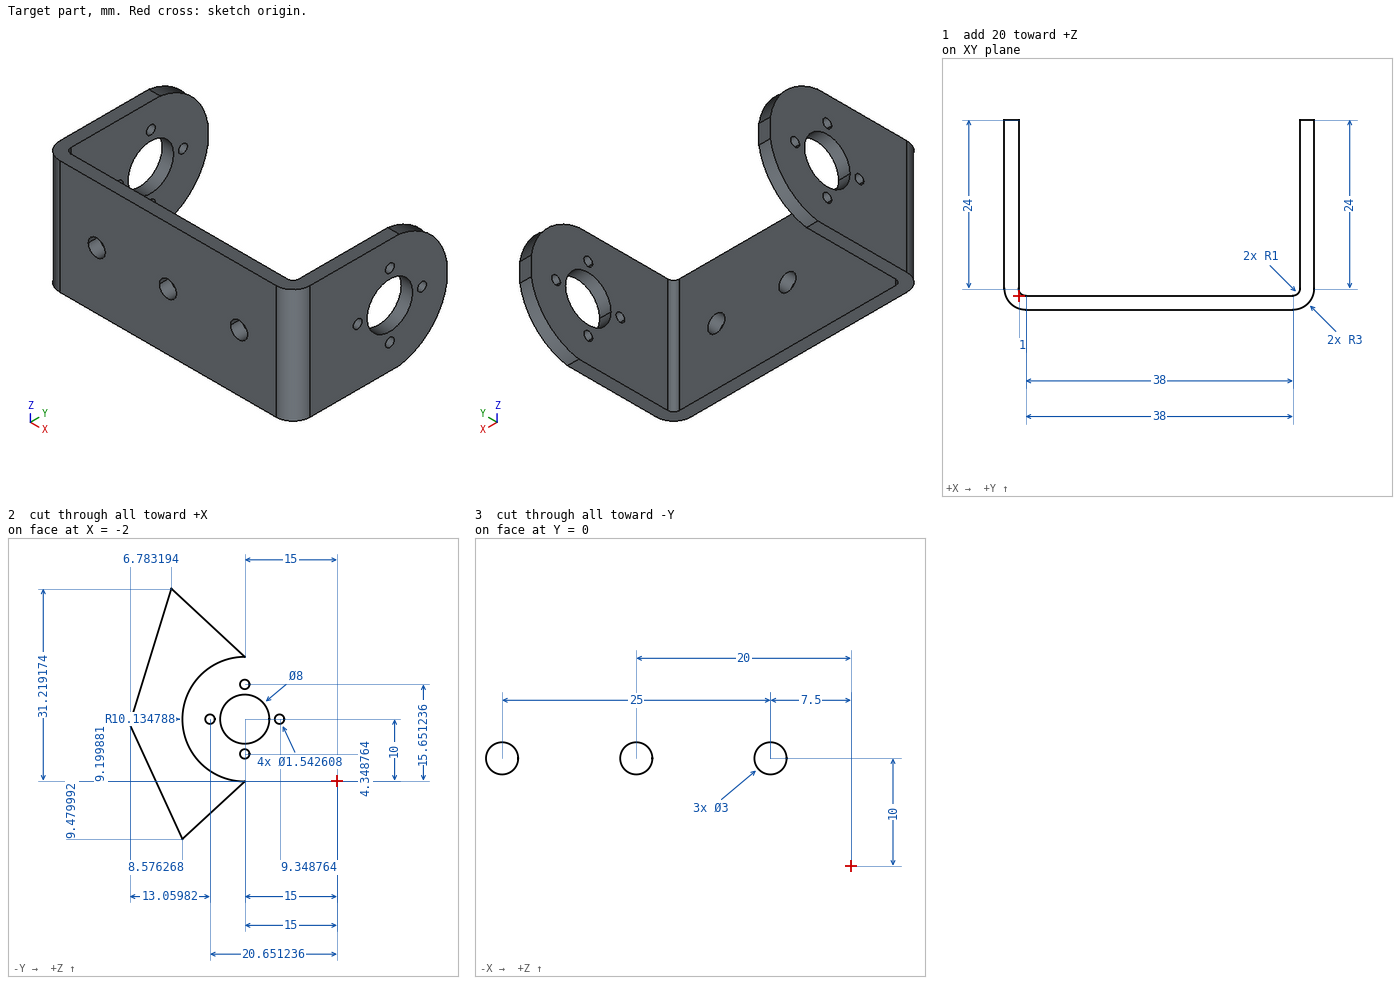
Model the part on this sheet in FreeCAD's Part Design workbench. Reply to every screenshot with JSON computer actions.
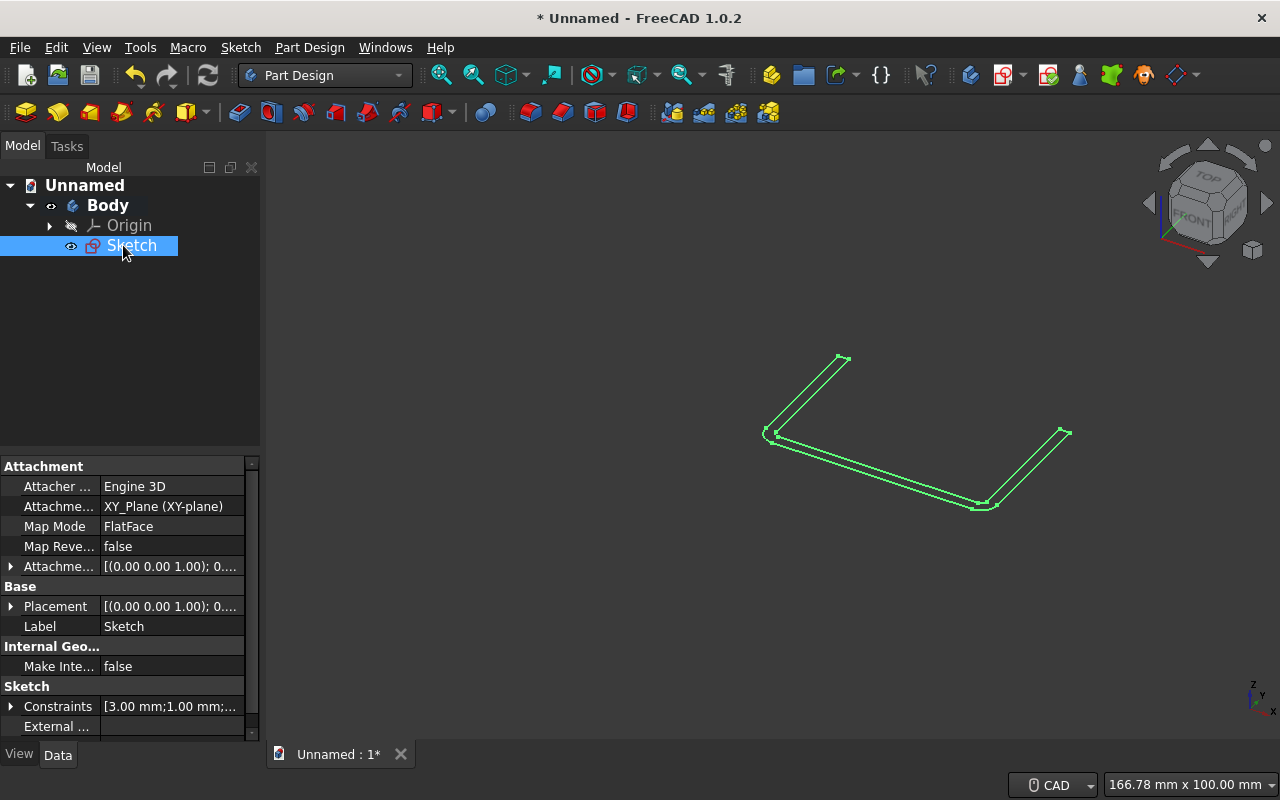
{"action": "left_click", "coordinate": [26, 112]}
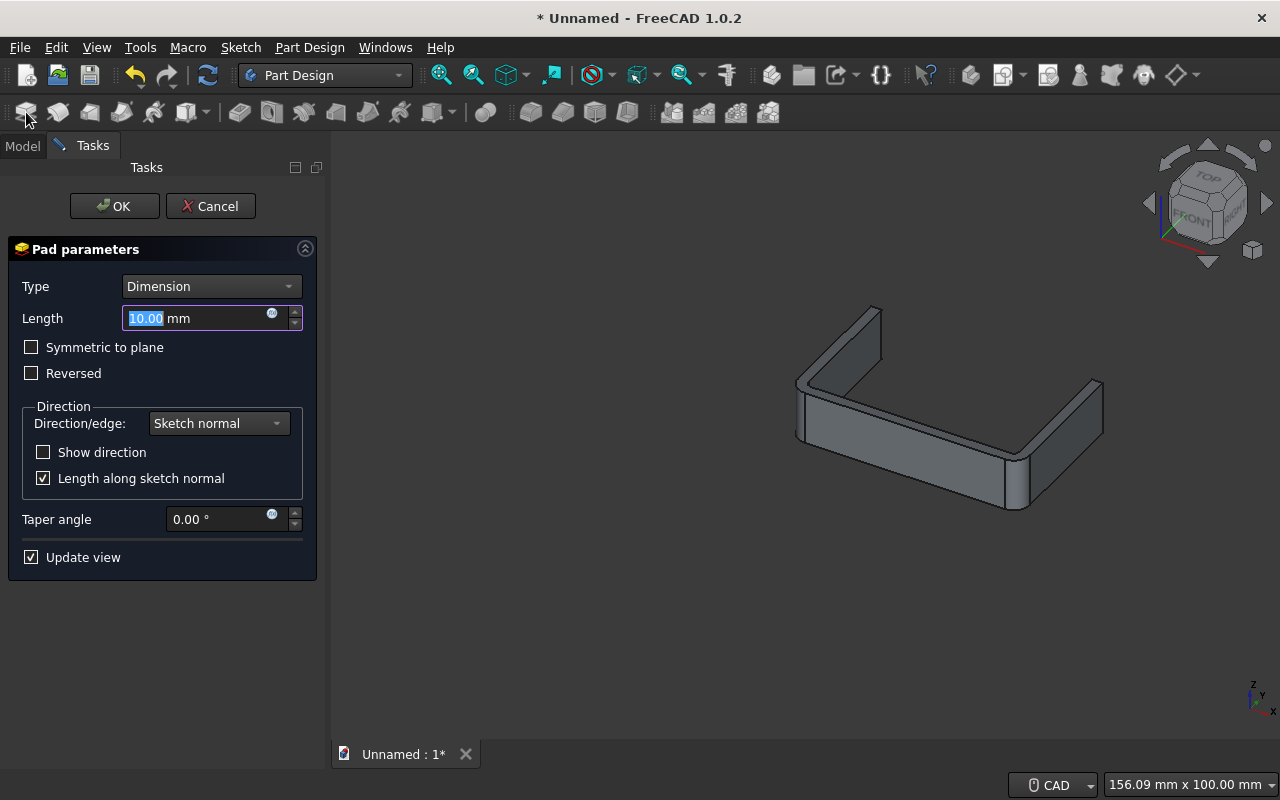
{"action": "type", "text": "20"}
{"action": "key", "text": "Tab"}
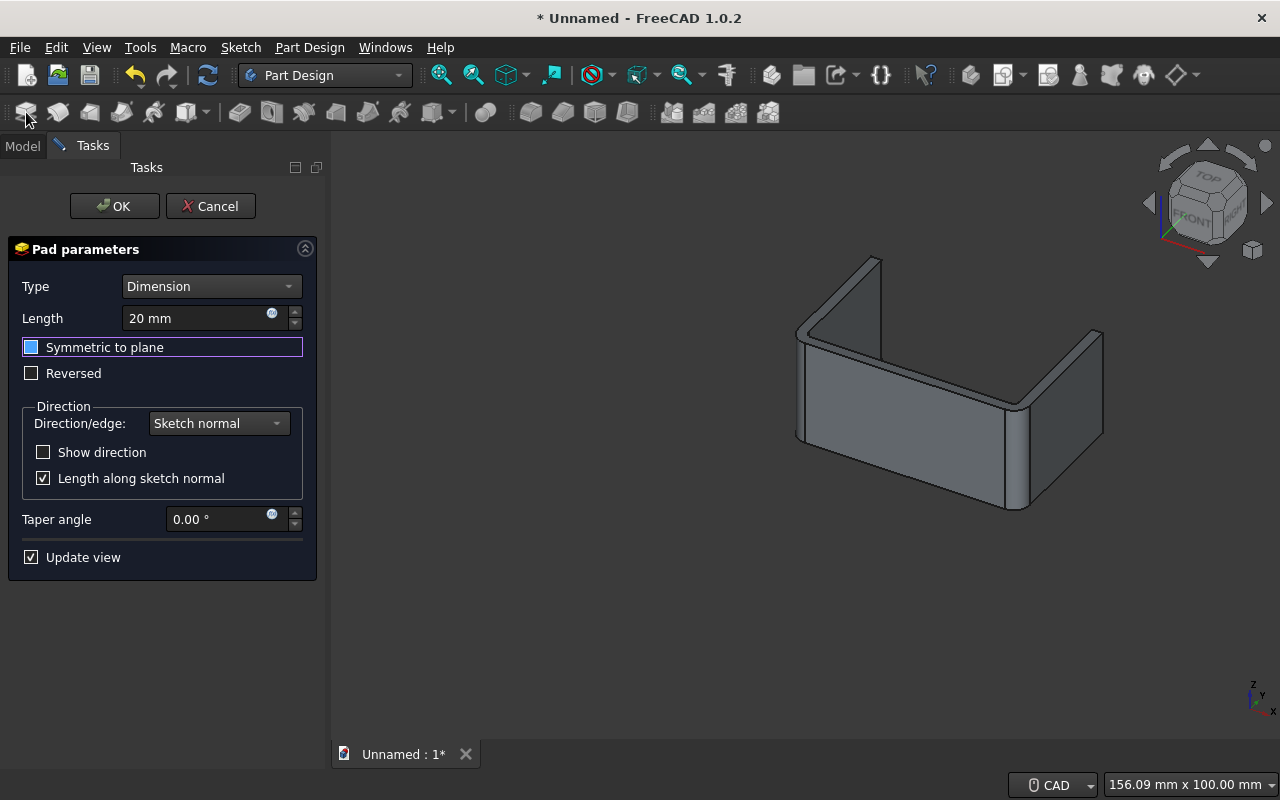
{"action": "left_click", "coordinate": [115, 206]}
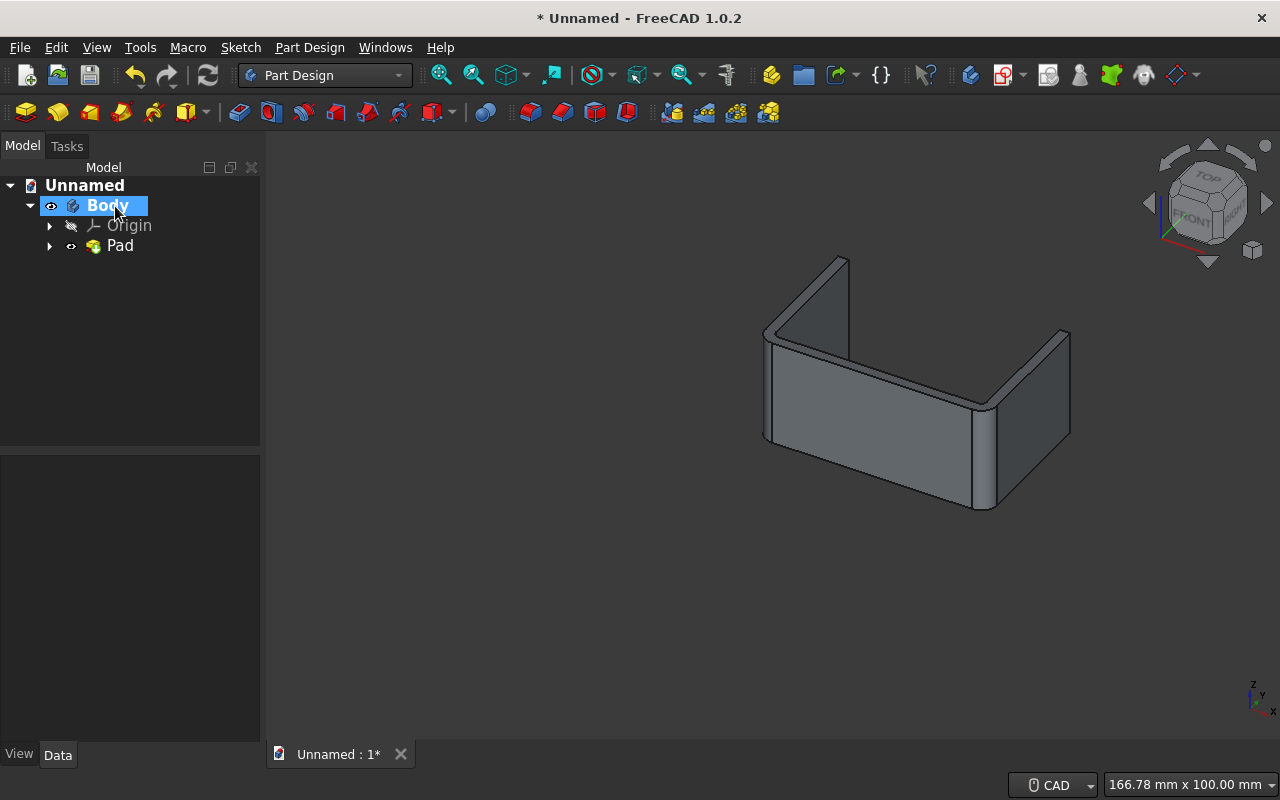
{"action": "left_click", "coordinate": [442, 76]}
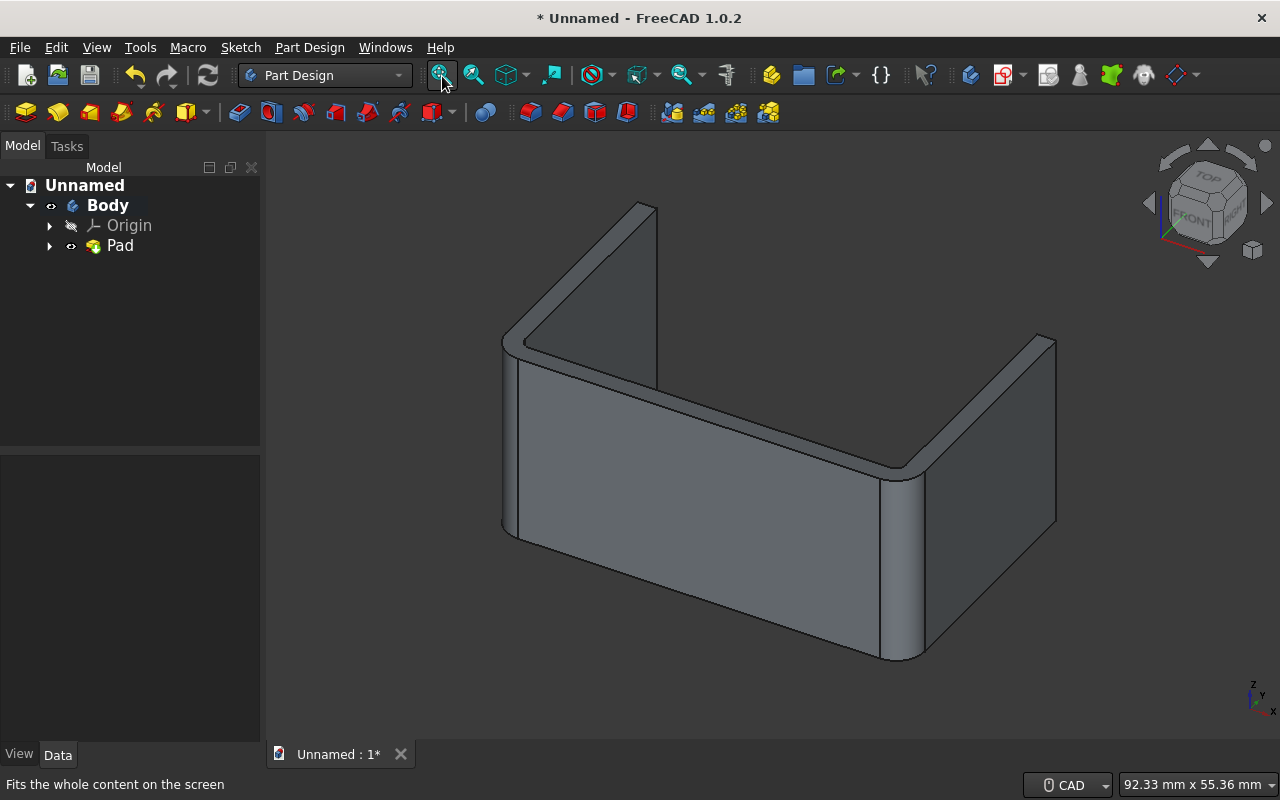
{"action": "key", "text": "6"}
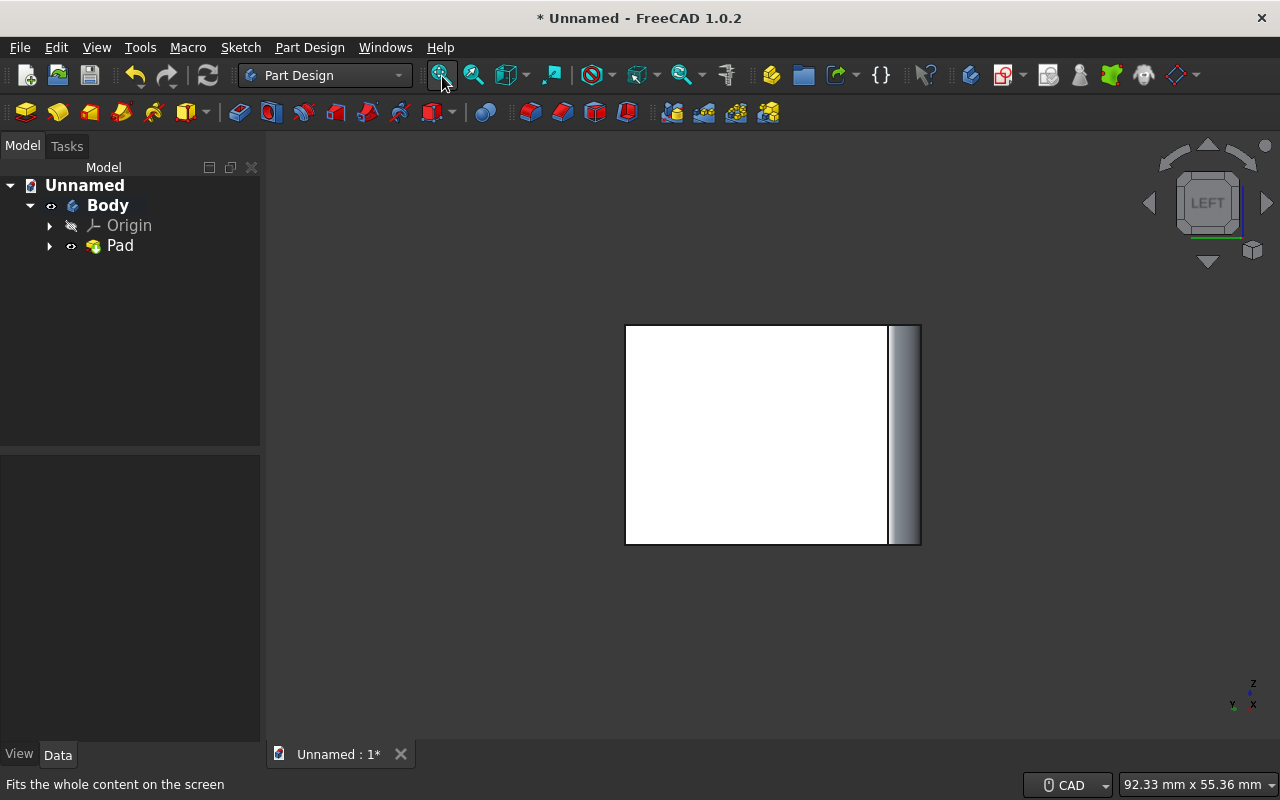
{"action": "left_click", "coordinate": [442, 76]}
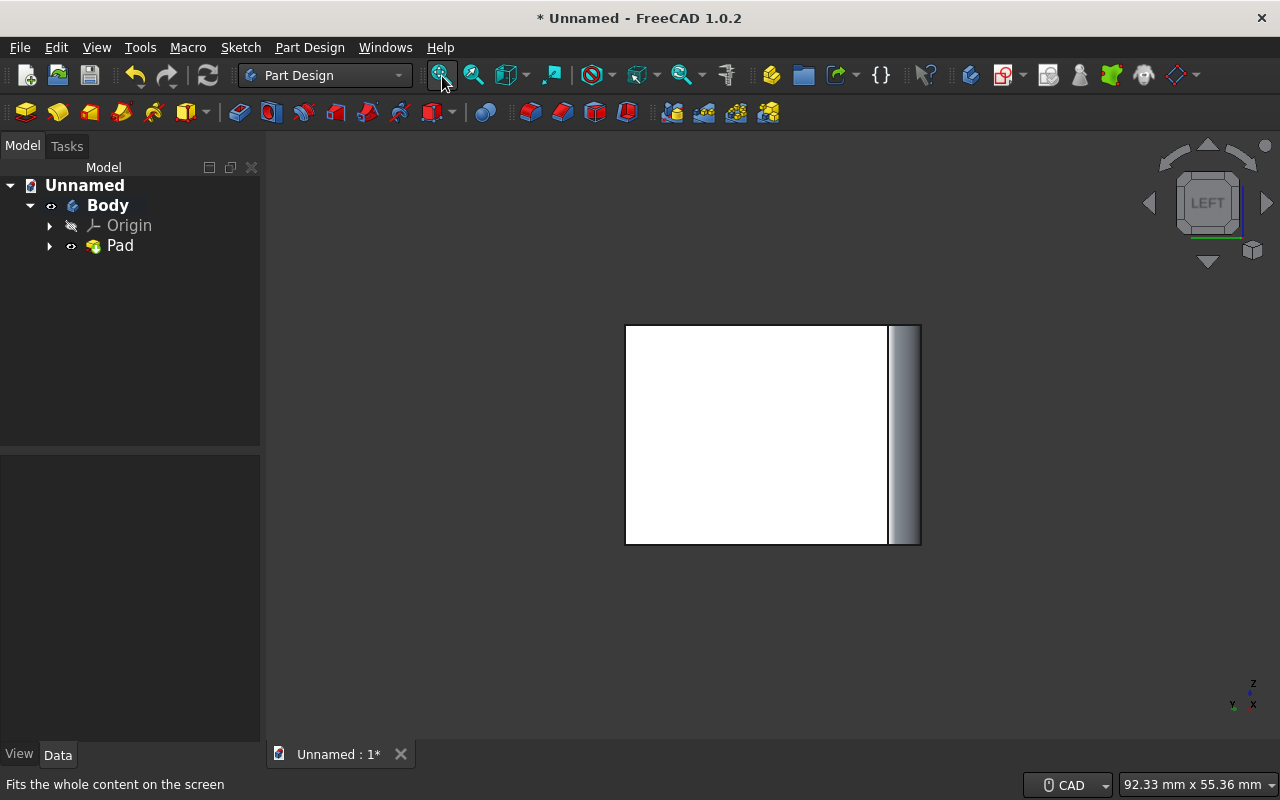
{"action": "left_click", "coordinate": [757, 434]}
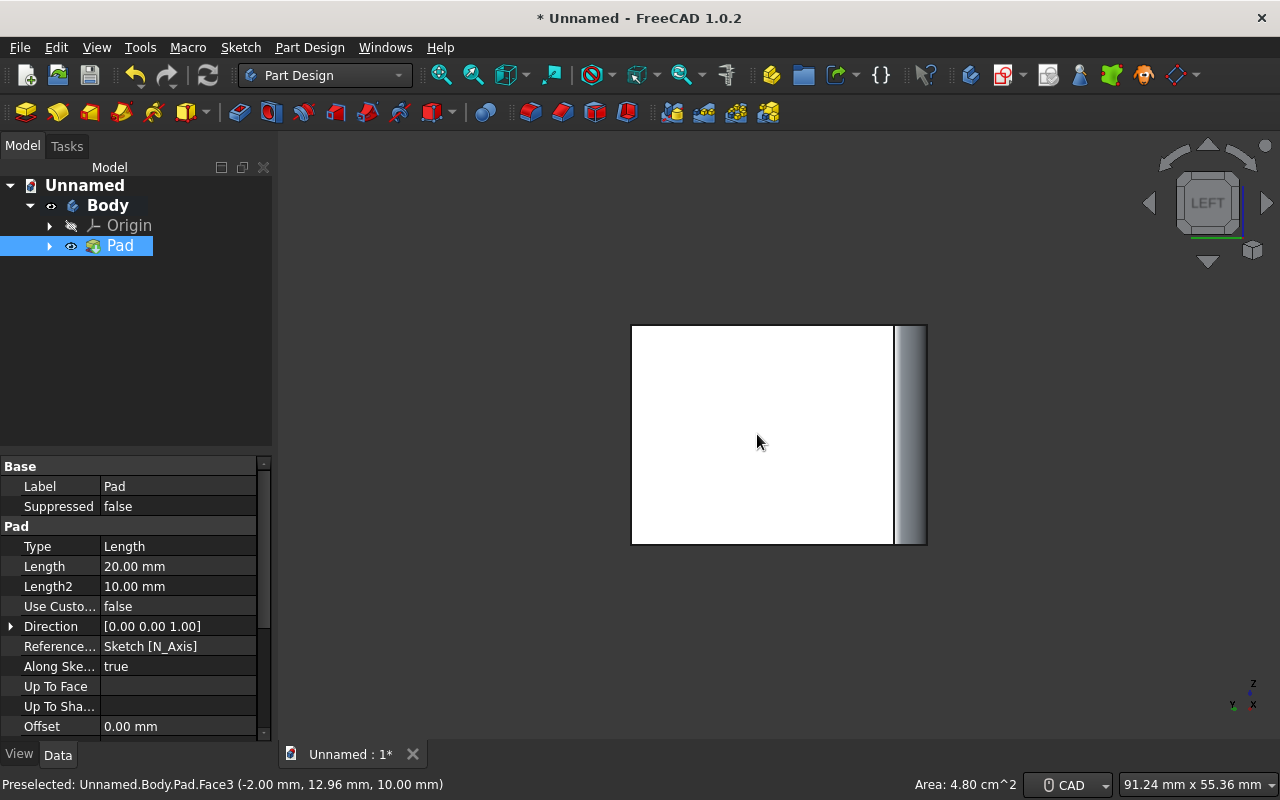
{"action": "left_click", "coordinate": [1004, 76]}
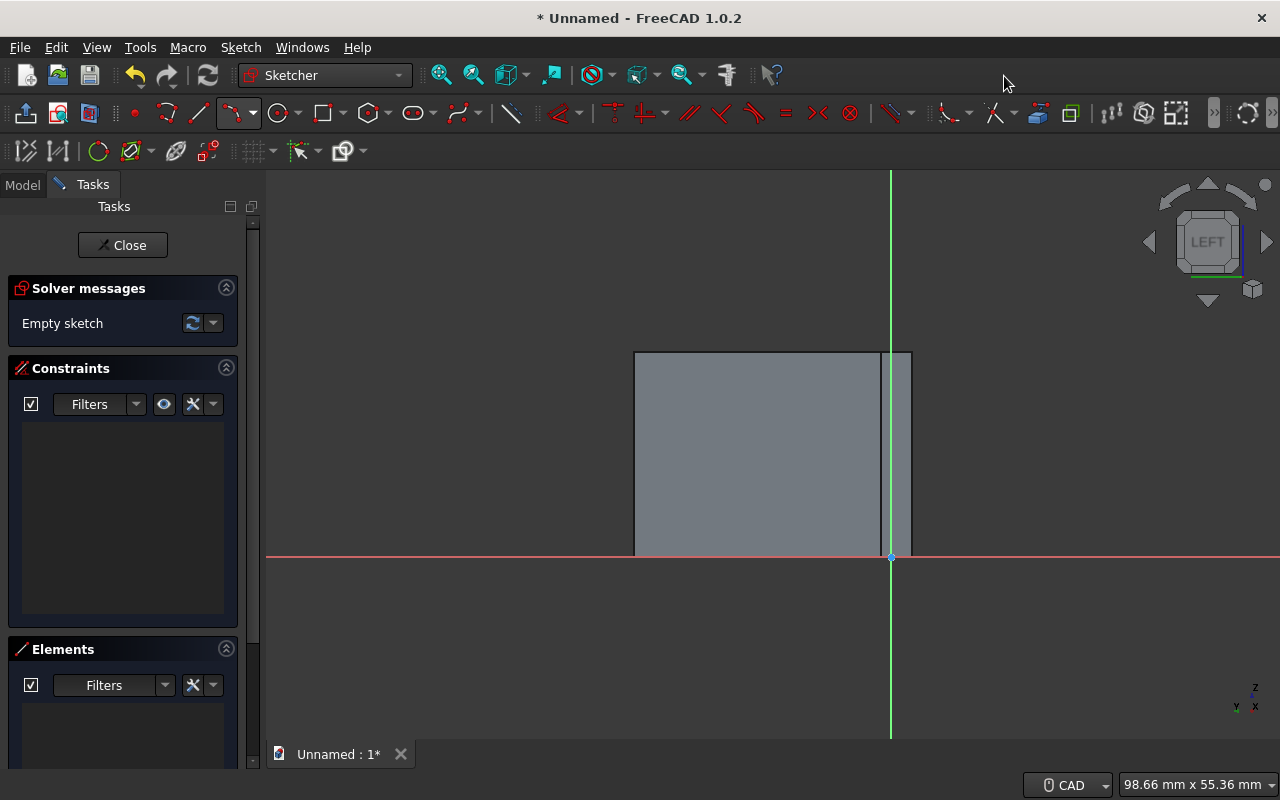
{"action": "key", "text": "g m"}